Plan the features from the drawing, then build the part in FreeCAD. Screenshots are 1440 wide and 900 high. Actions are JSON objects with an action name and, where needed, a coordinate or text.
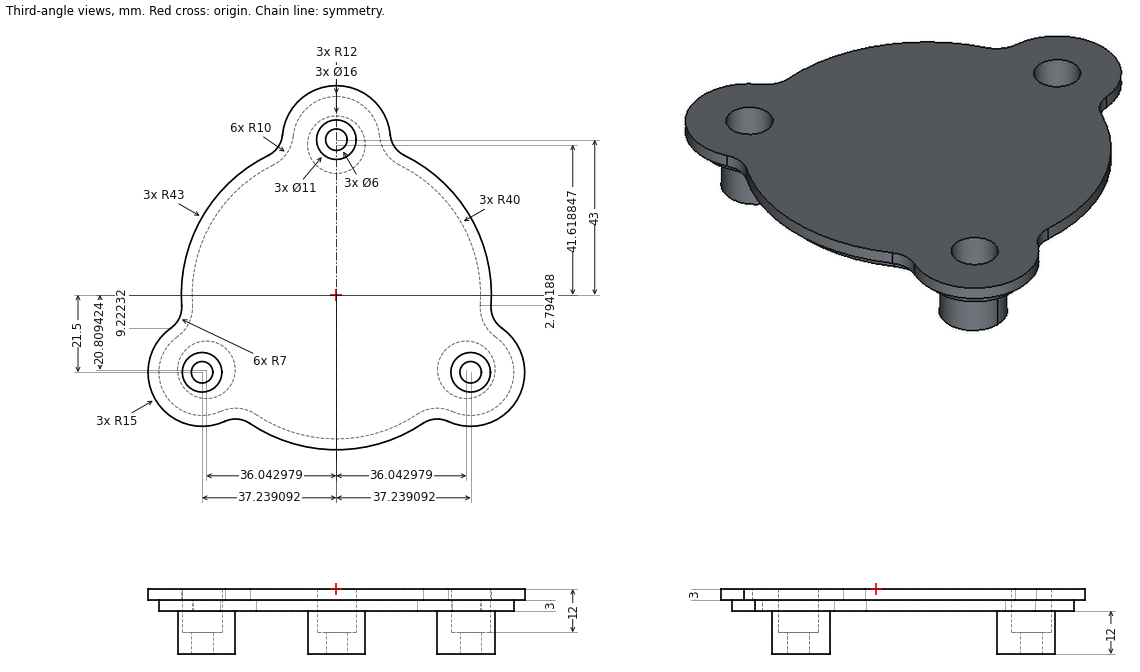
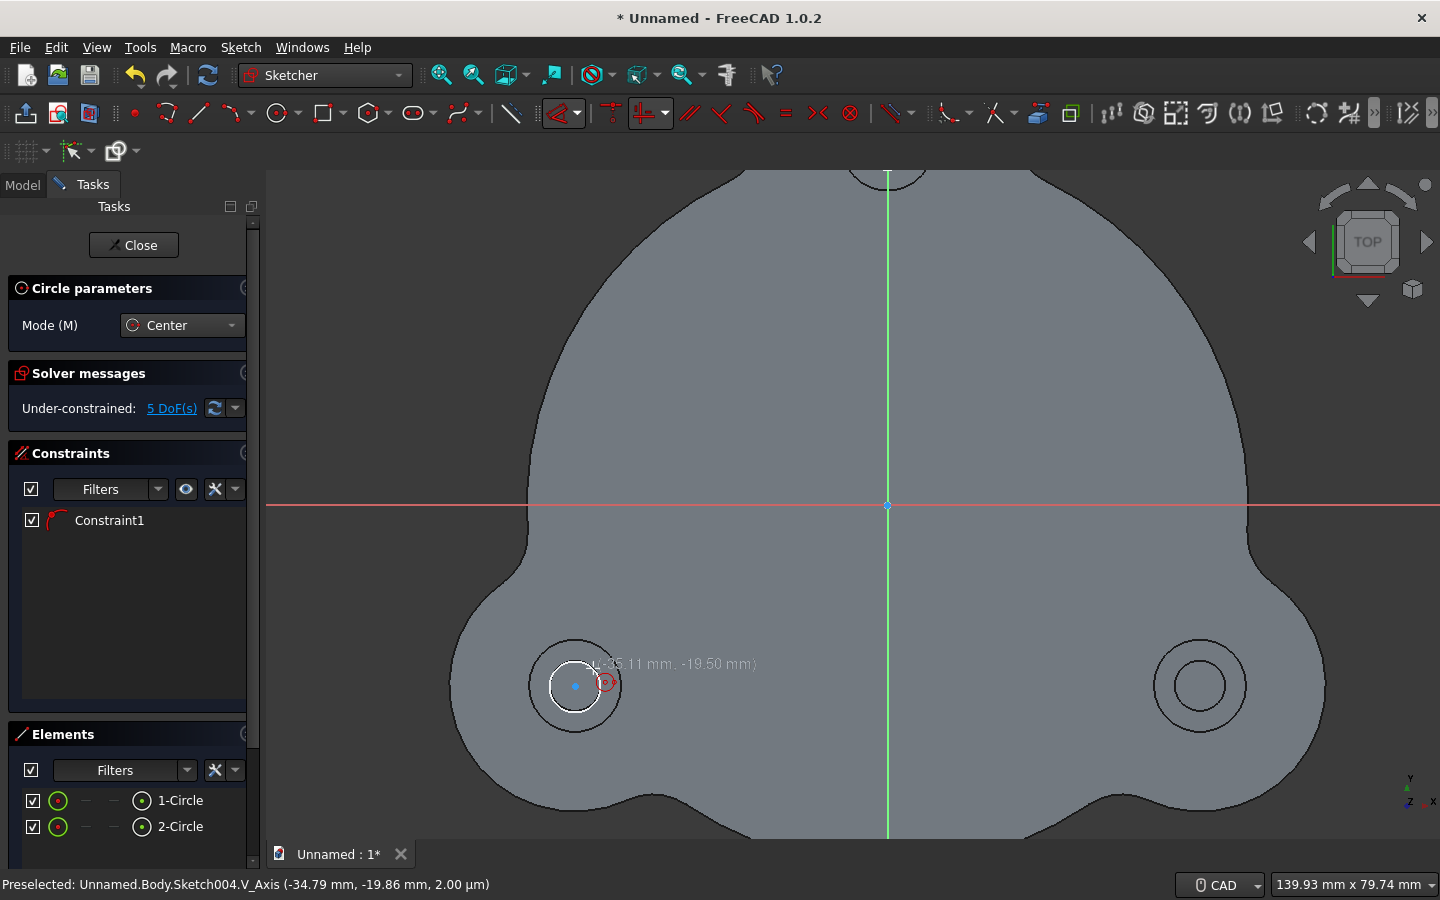
{"action": "left_click", "coordinate": [1200, 686]}
{"action": "left_click", "coordinate": [1218, 668]}
{"action": "key", "text": "Escape"}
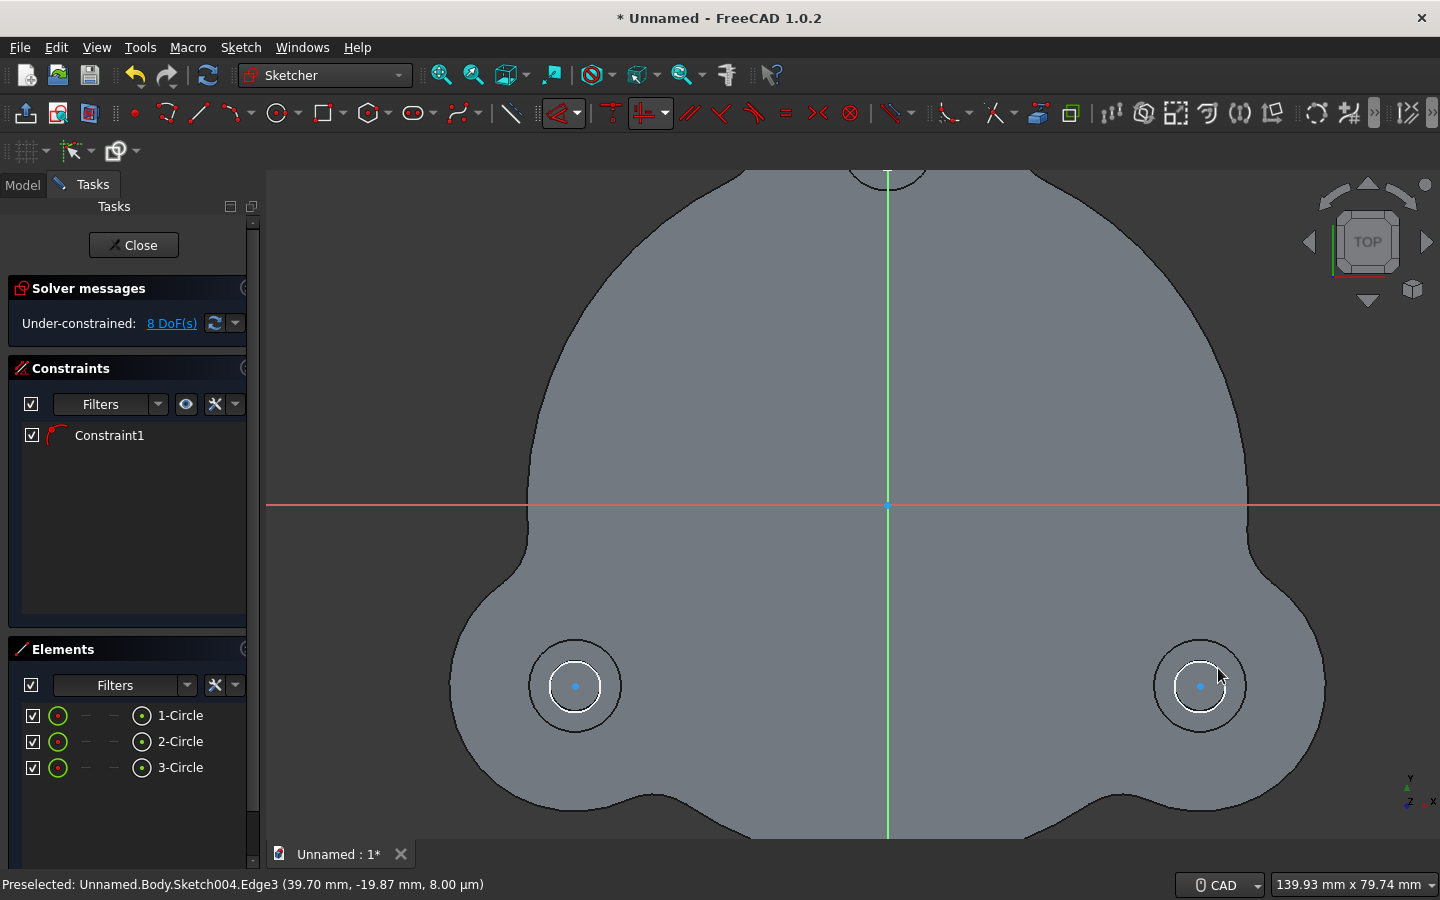
{"action": "scroll", "coordinate": [575, 686], "scroll_direction": "down", "scroll_amount": 2}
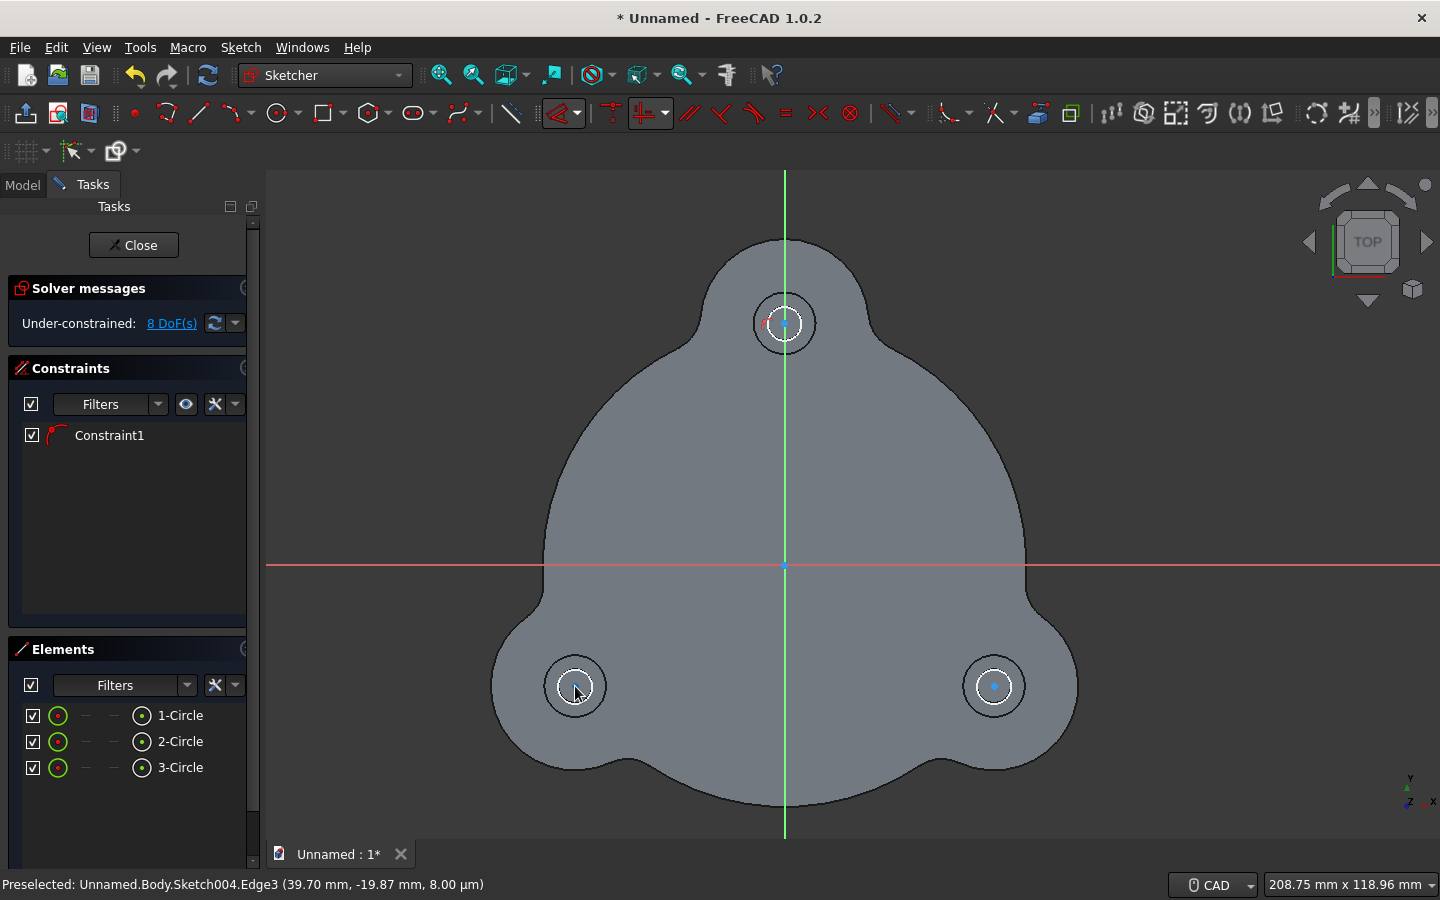
{"action": "left_click", "coordinate": [796, 312]}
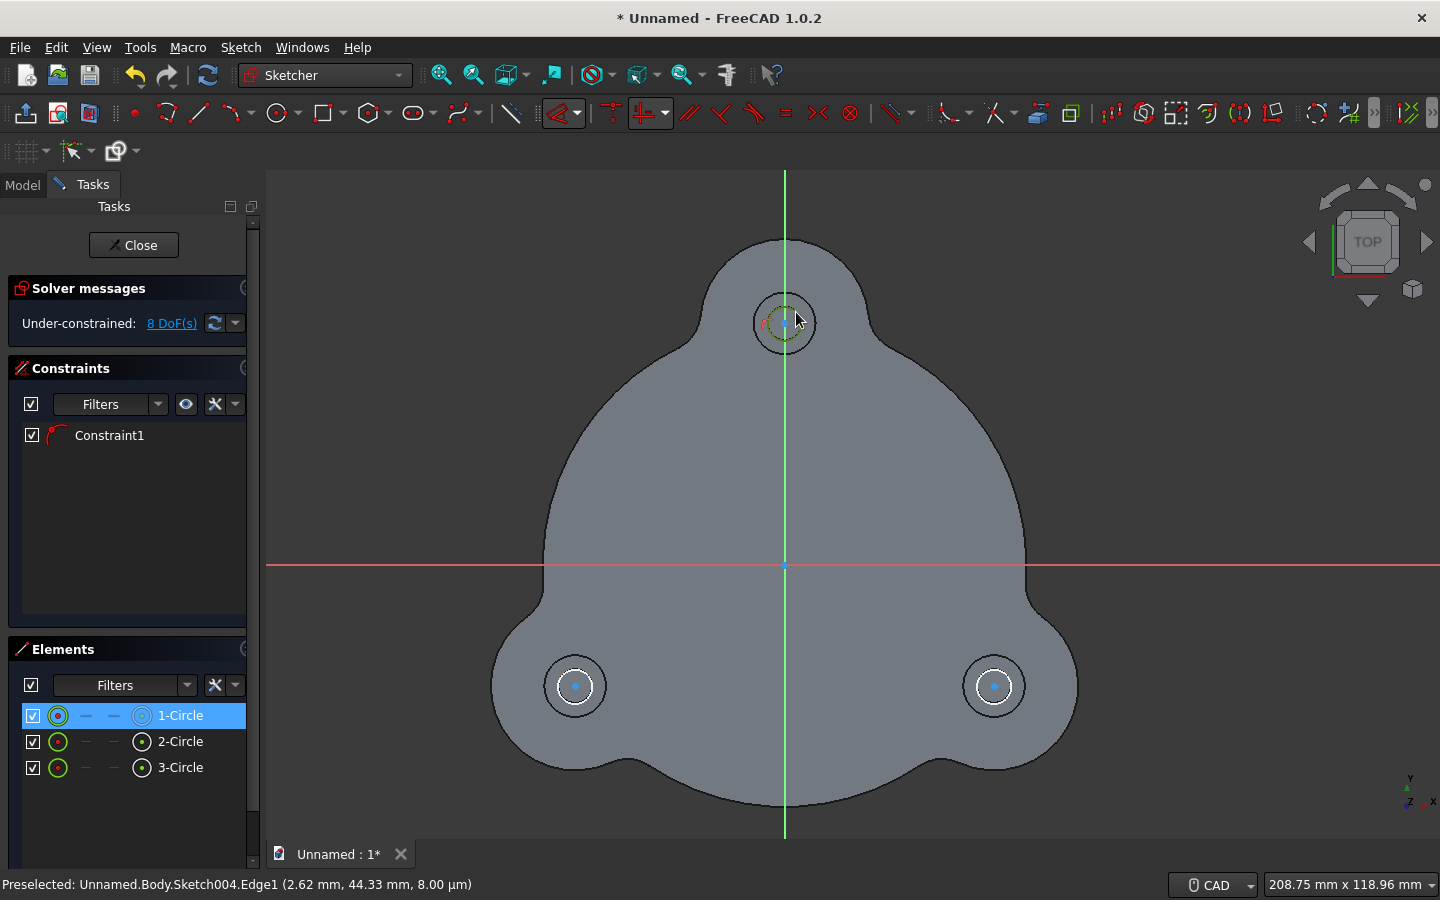
{"action": "left_click", "coordinate": [587, 675]}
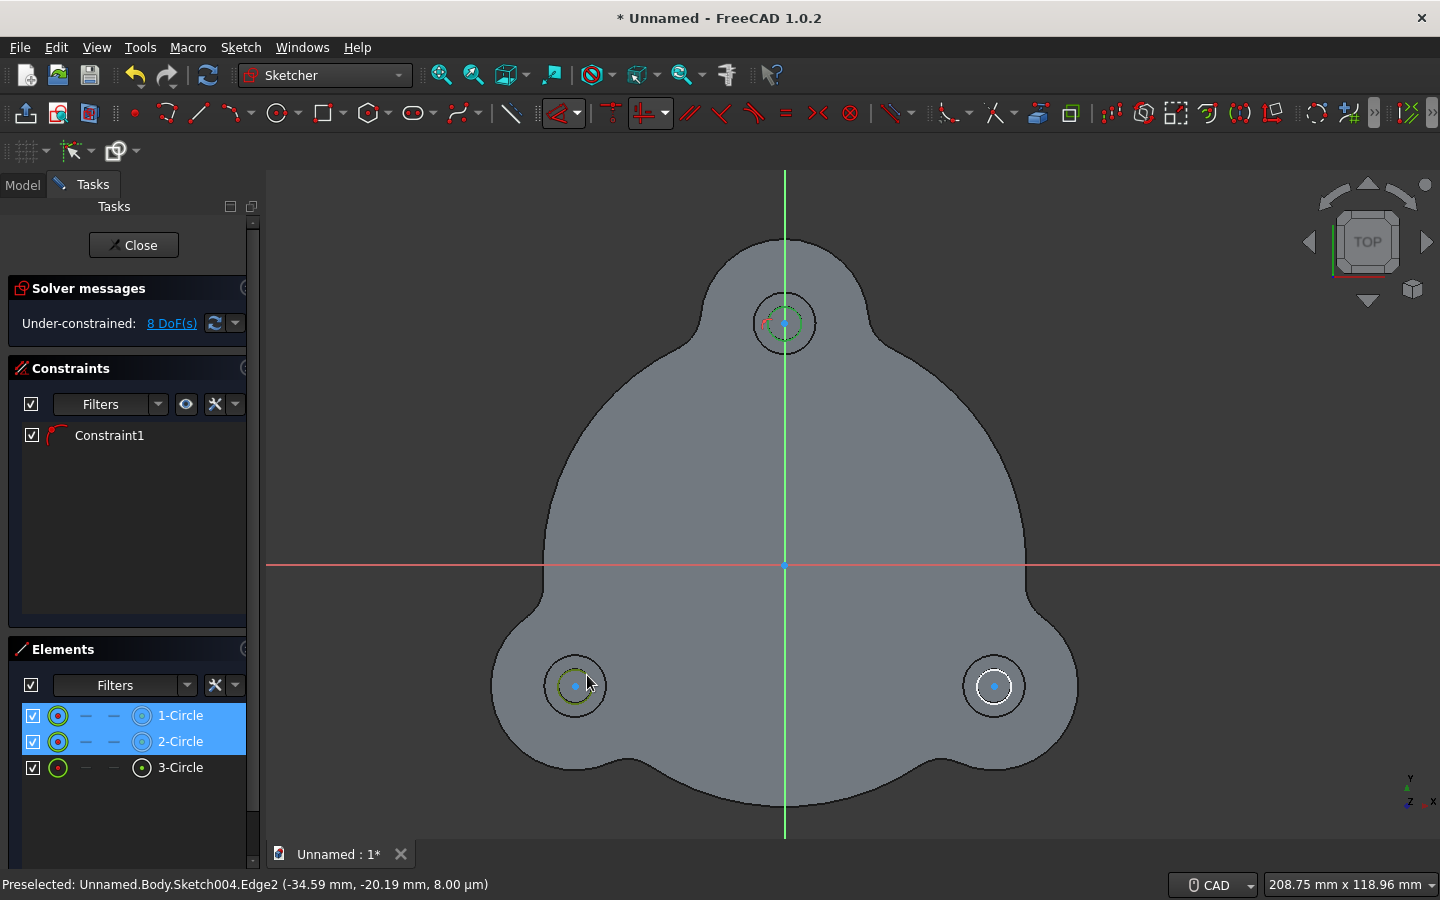
{"action": "left_click", "coordinate": [1006, 675]}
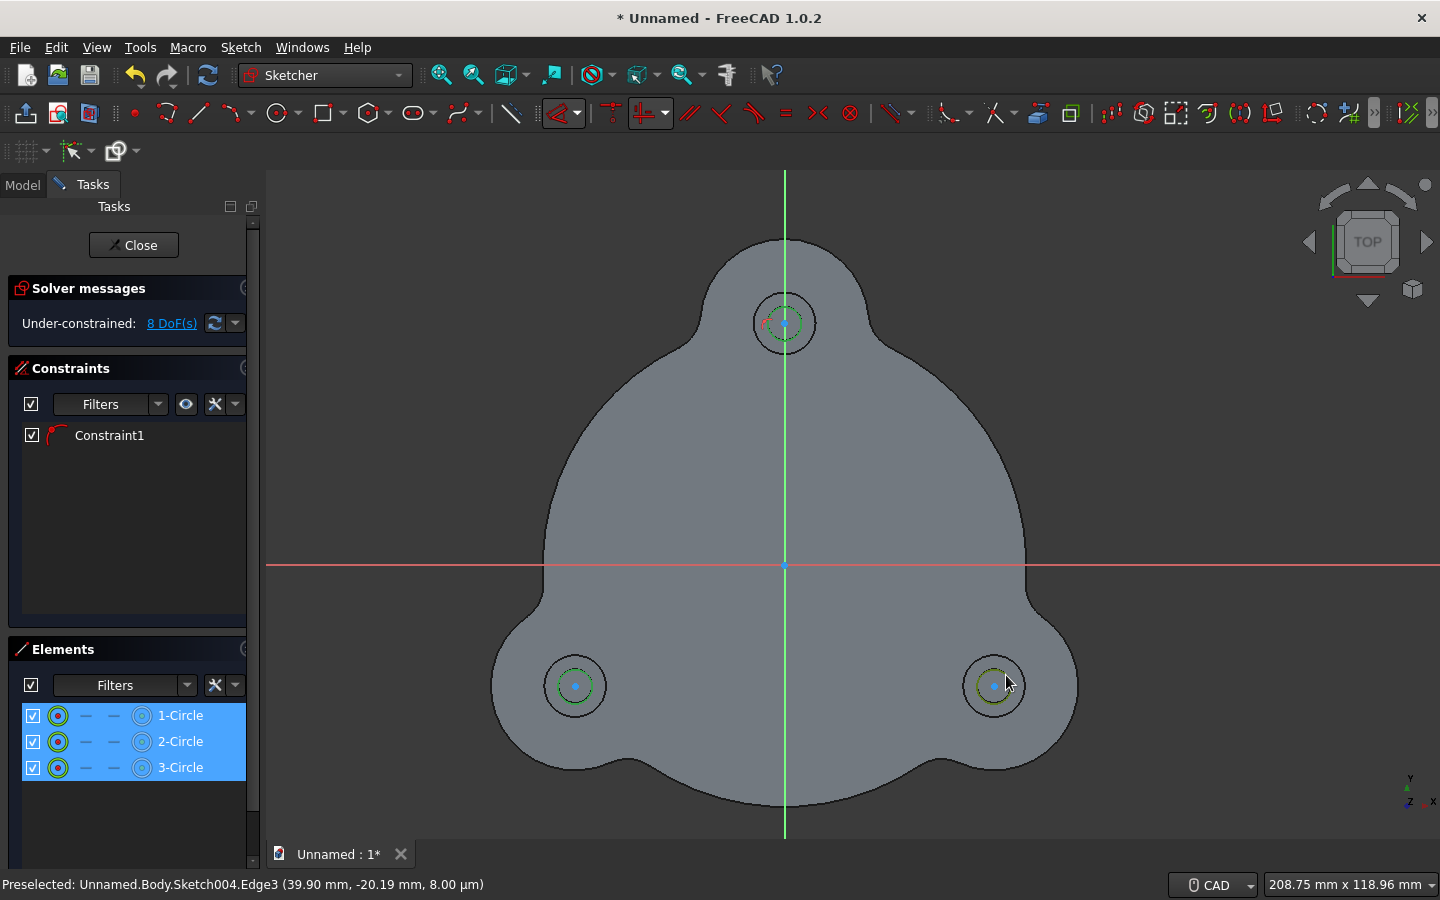
{"action": "left_click", "coordinate": [786, 114]}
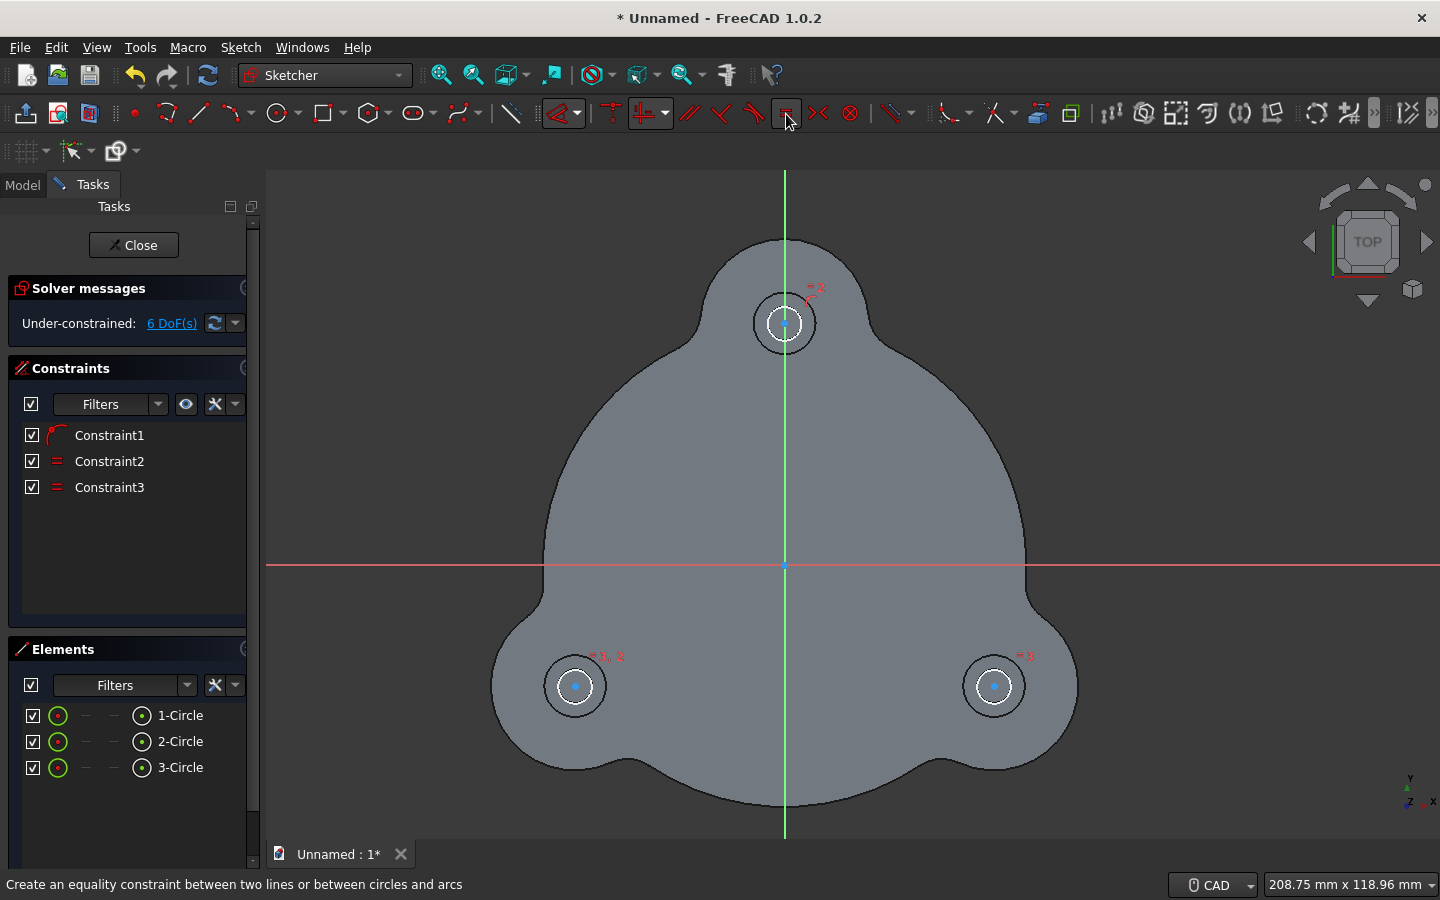
{"action": "left_click", "coordinate": [575, 687]}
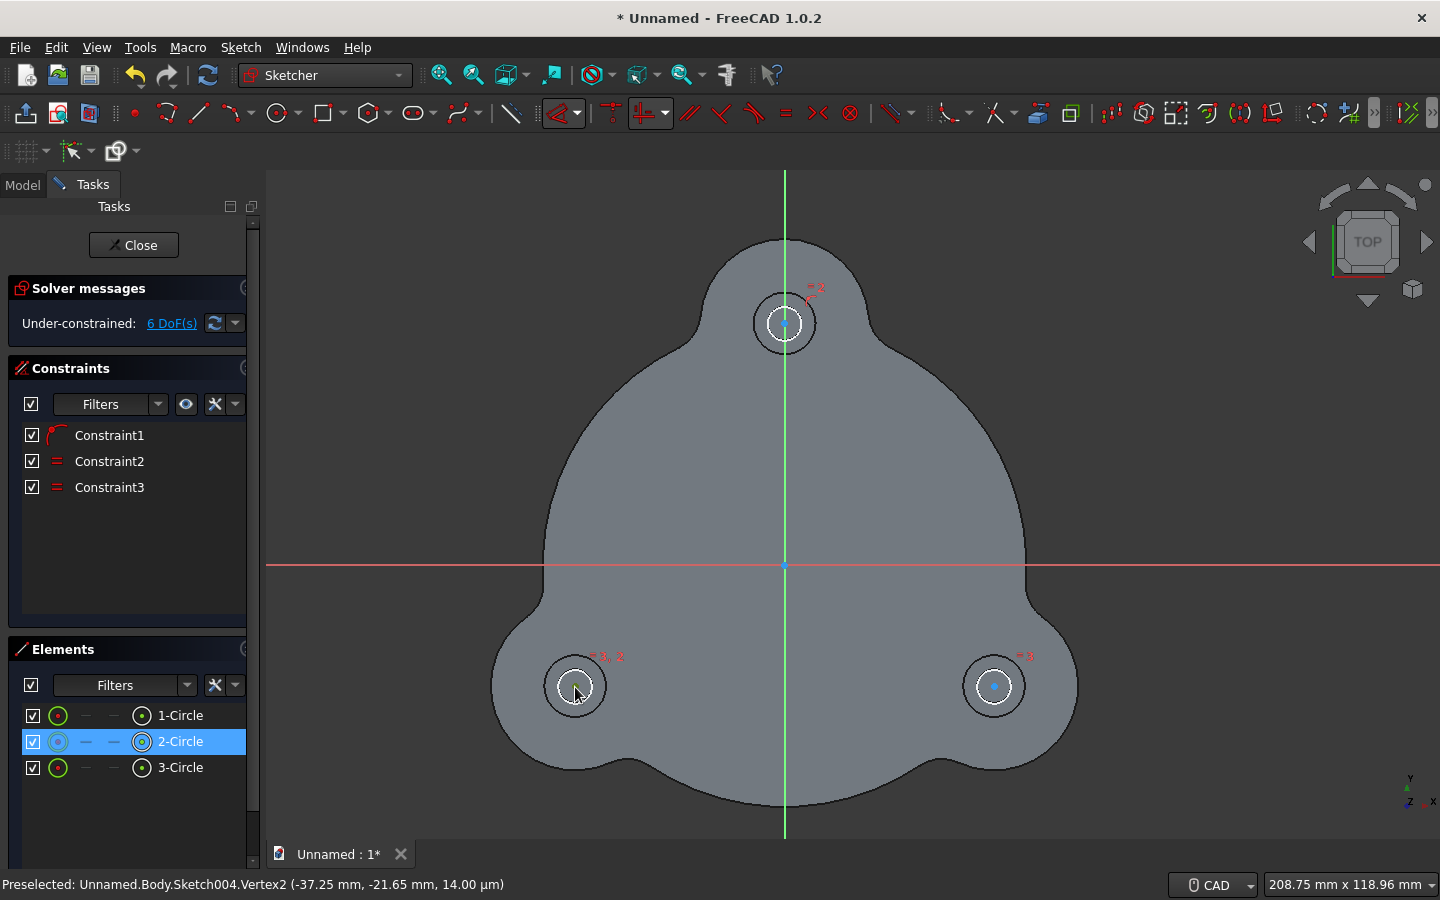
{"action": "left_click", "coordinate": [994, 687]}